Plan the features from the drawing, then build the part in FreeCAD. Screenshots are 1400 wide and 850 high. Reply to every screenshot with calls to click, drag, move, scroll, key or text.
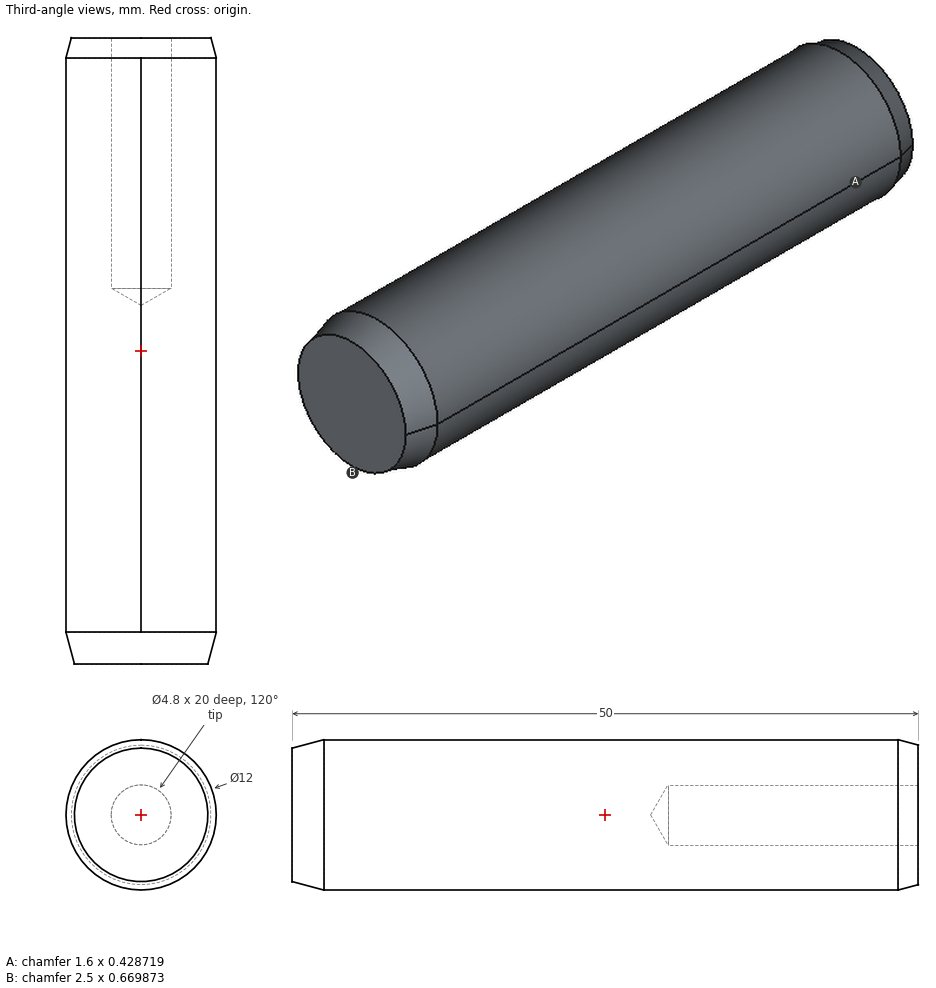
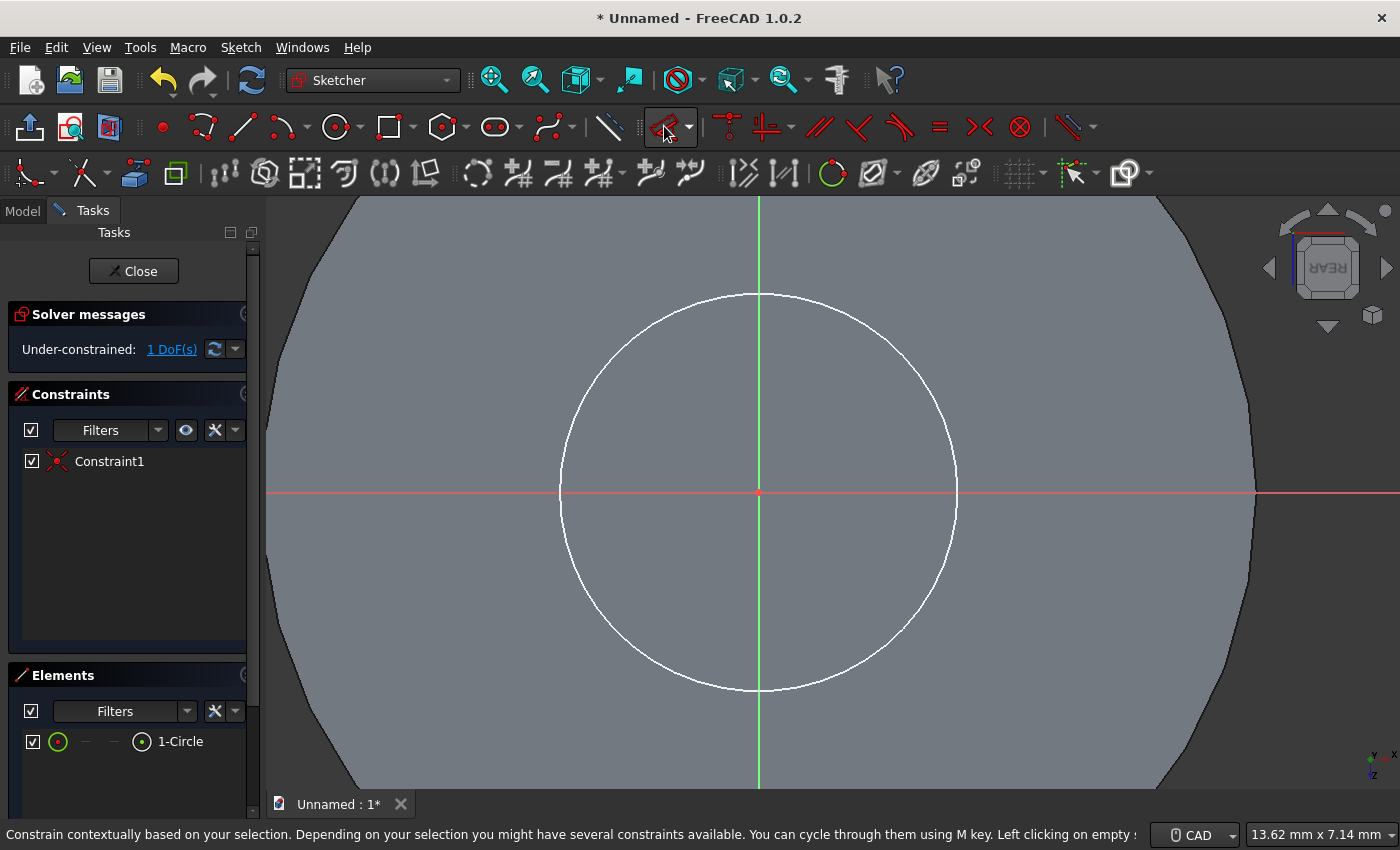
click(899, 352)
click(922, 329)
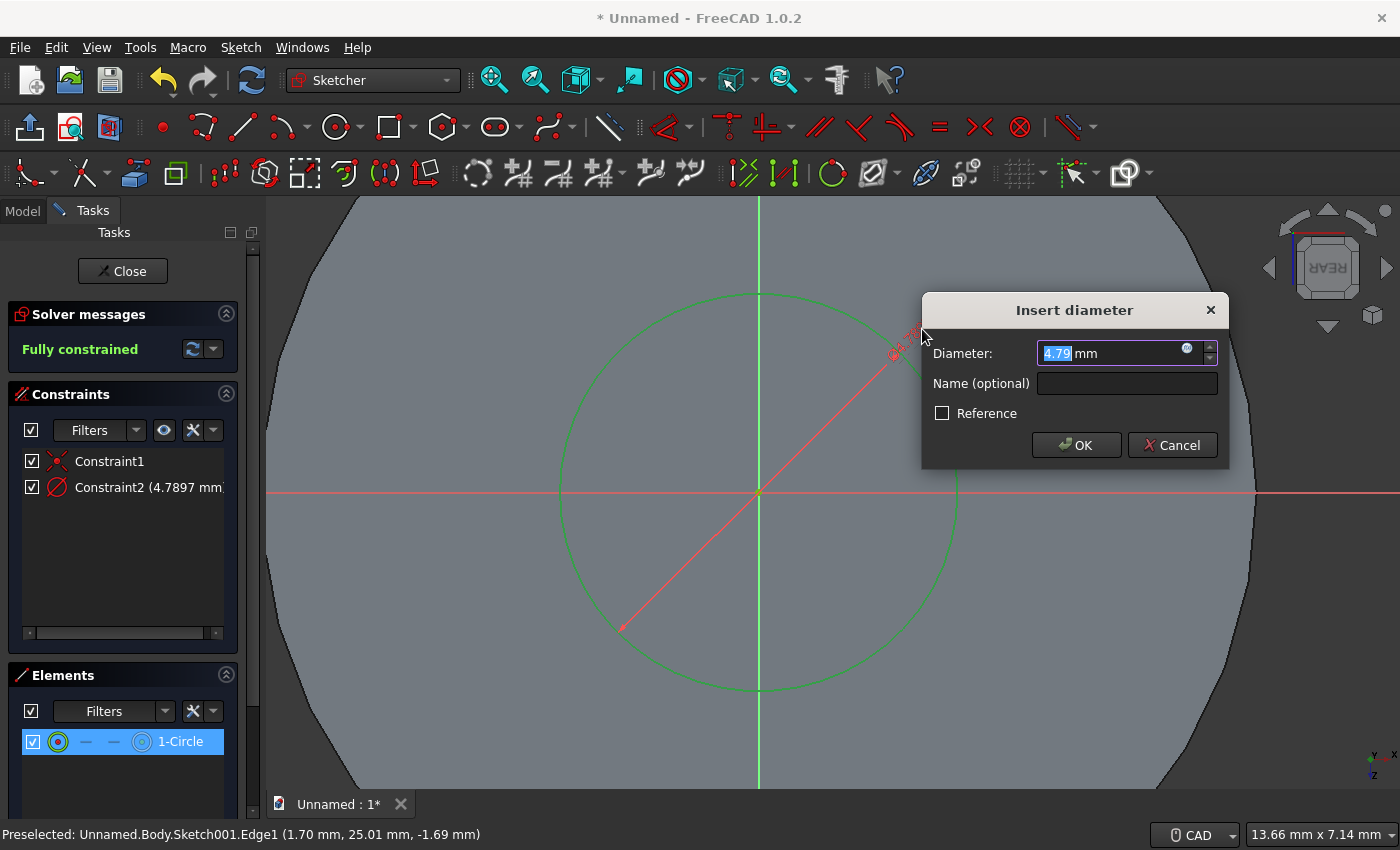
text(4.8)
key(Return)
key(Escape)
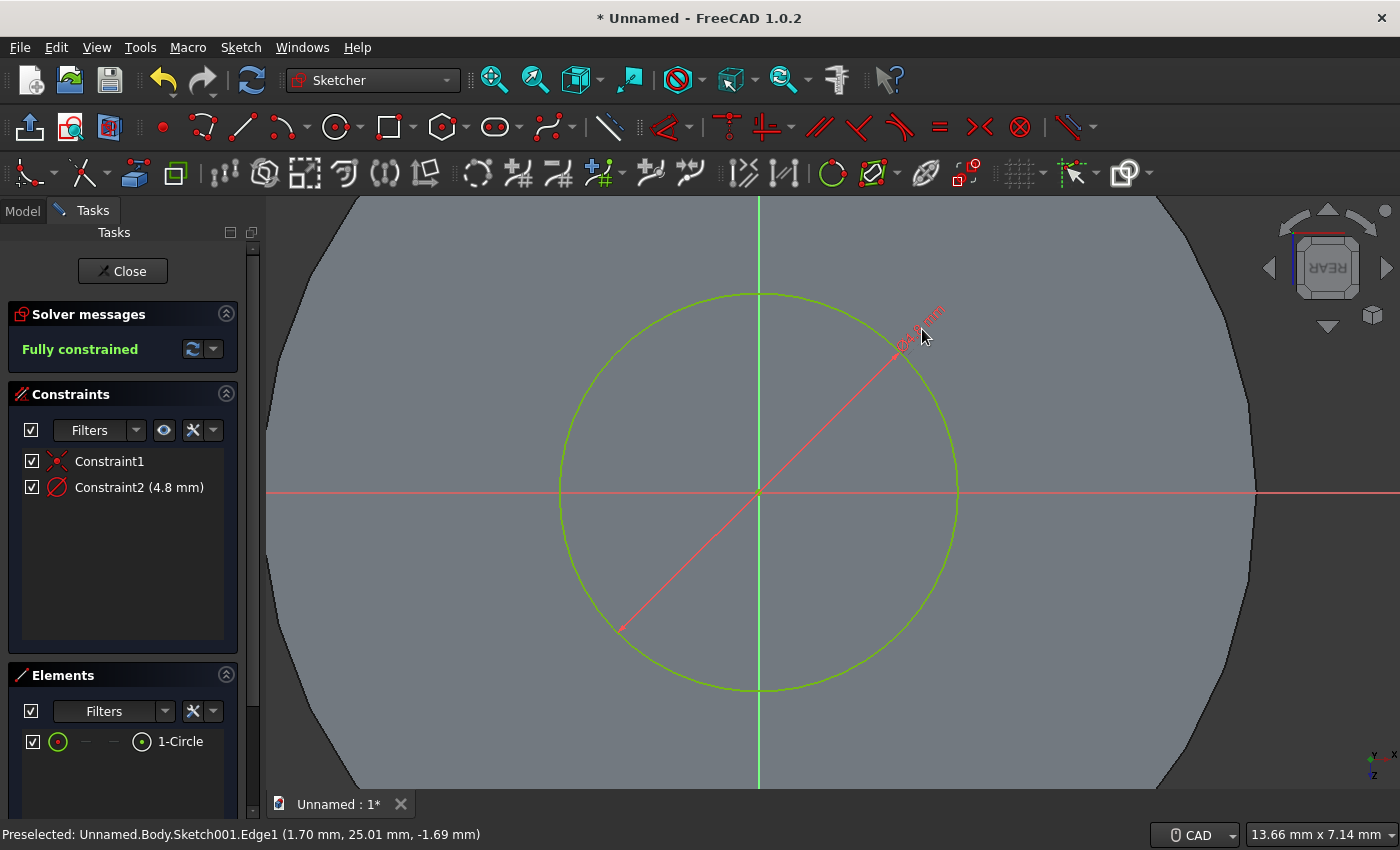
click(123, 271)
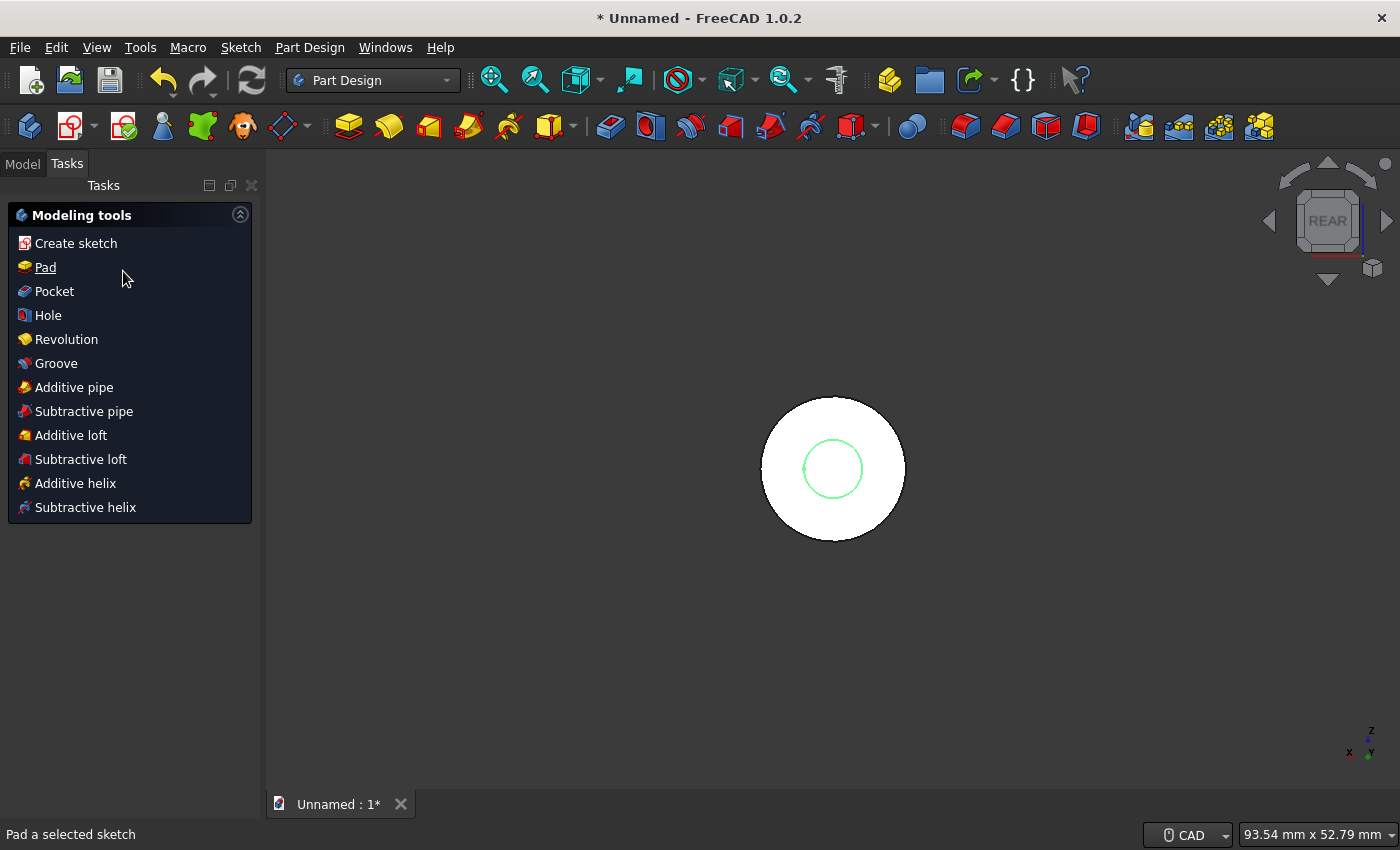
click(652, 126)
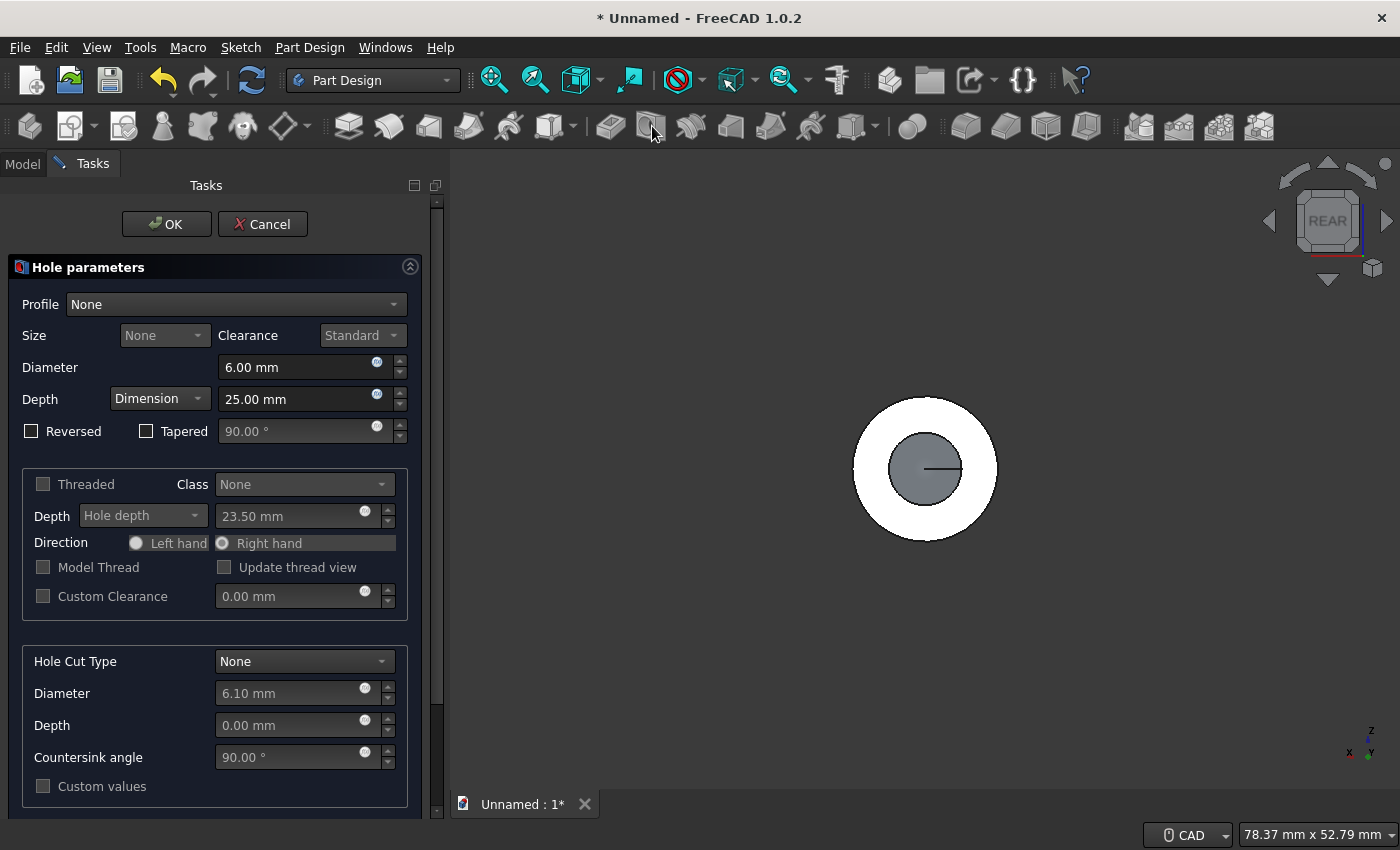
triple_click(305, 367)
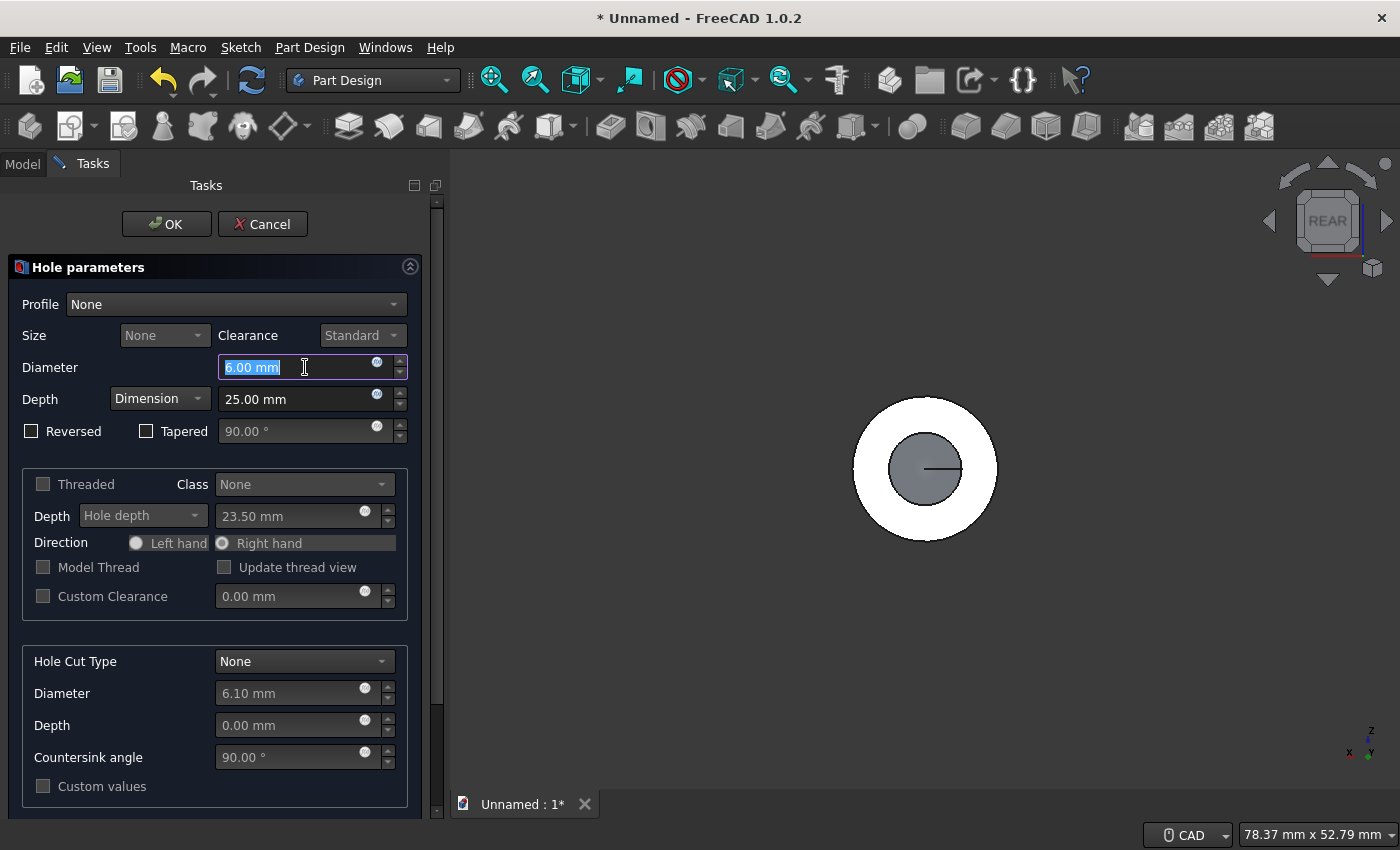
text(4.8)
key(Tab)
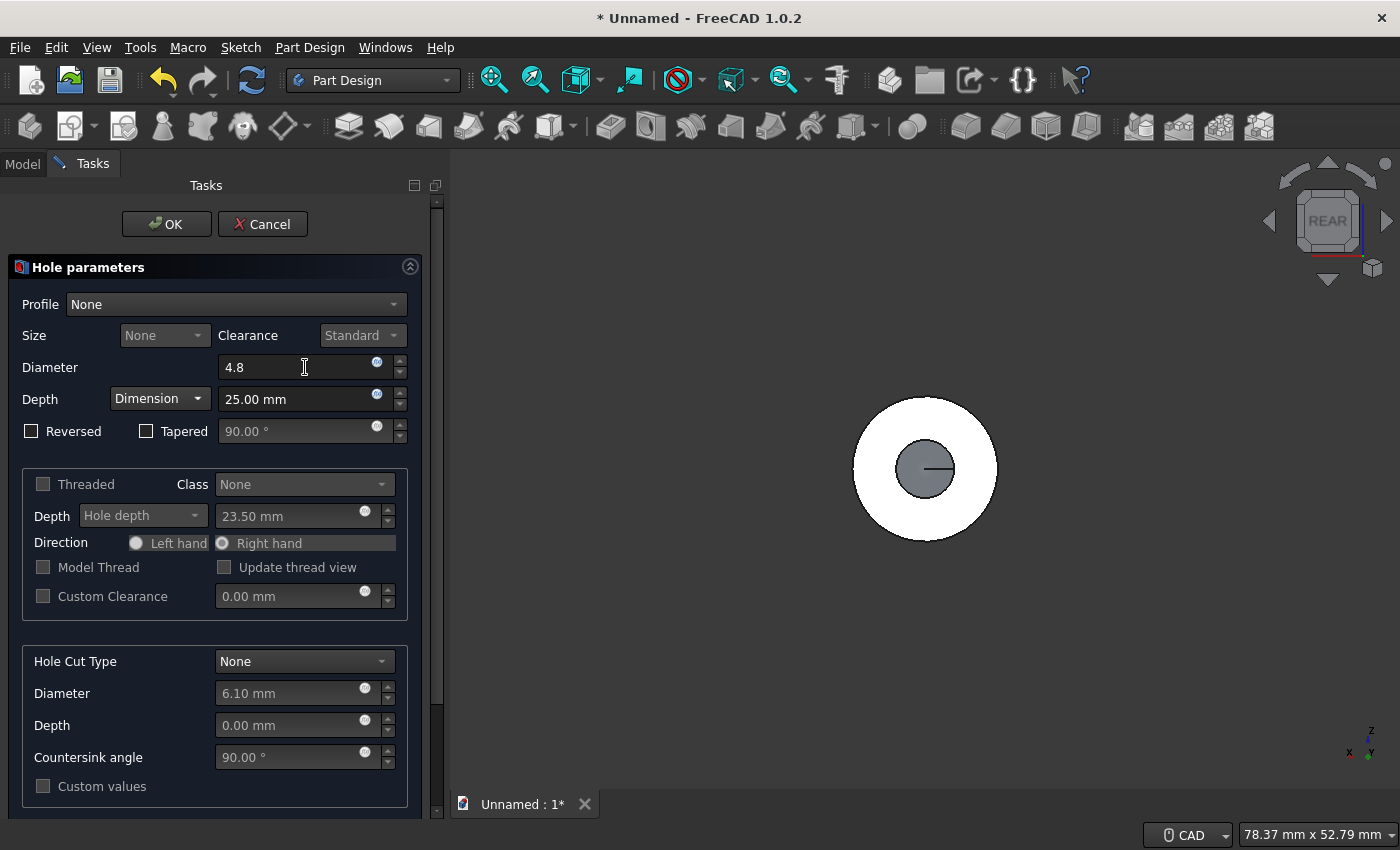
triple_click(305, 399)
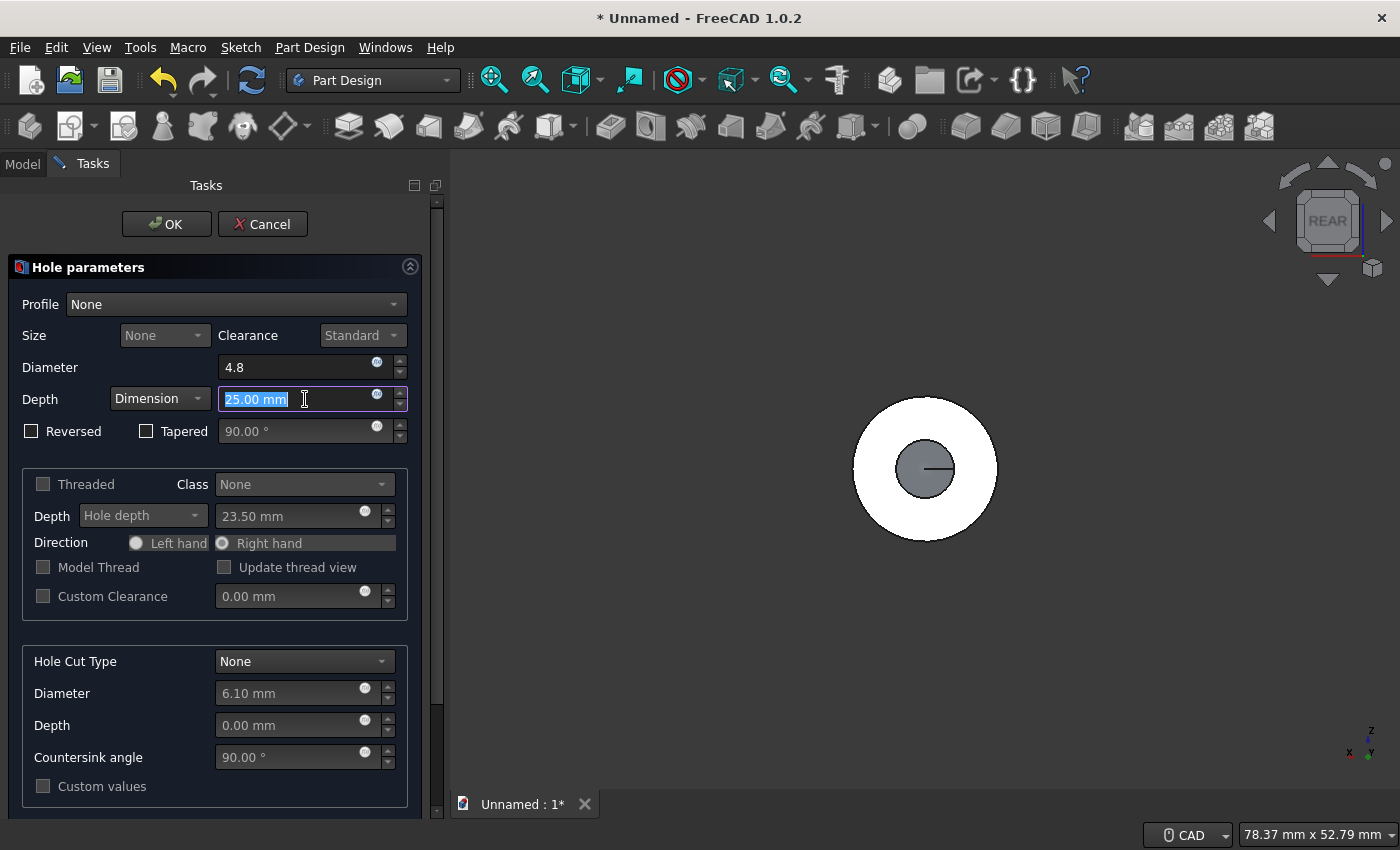
text(20)
key(Tab)